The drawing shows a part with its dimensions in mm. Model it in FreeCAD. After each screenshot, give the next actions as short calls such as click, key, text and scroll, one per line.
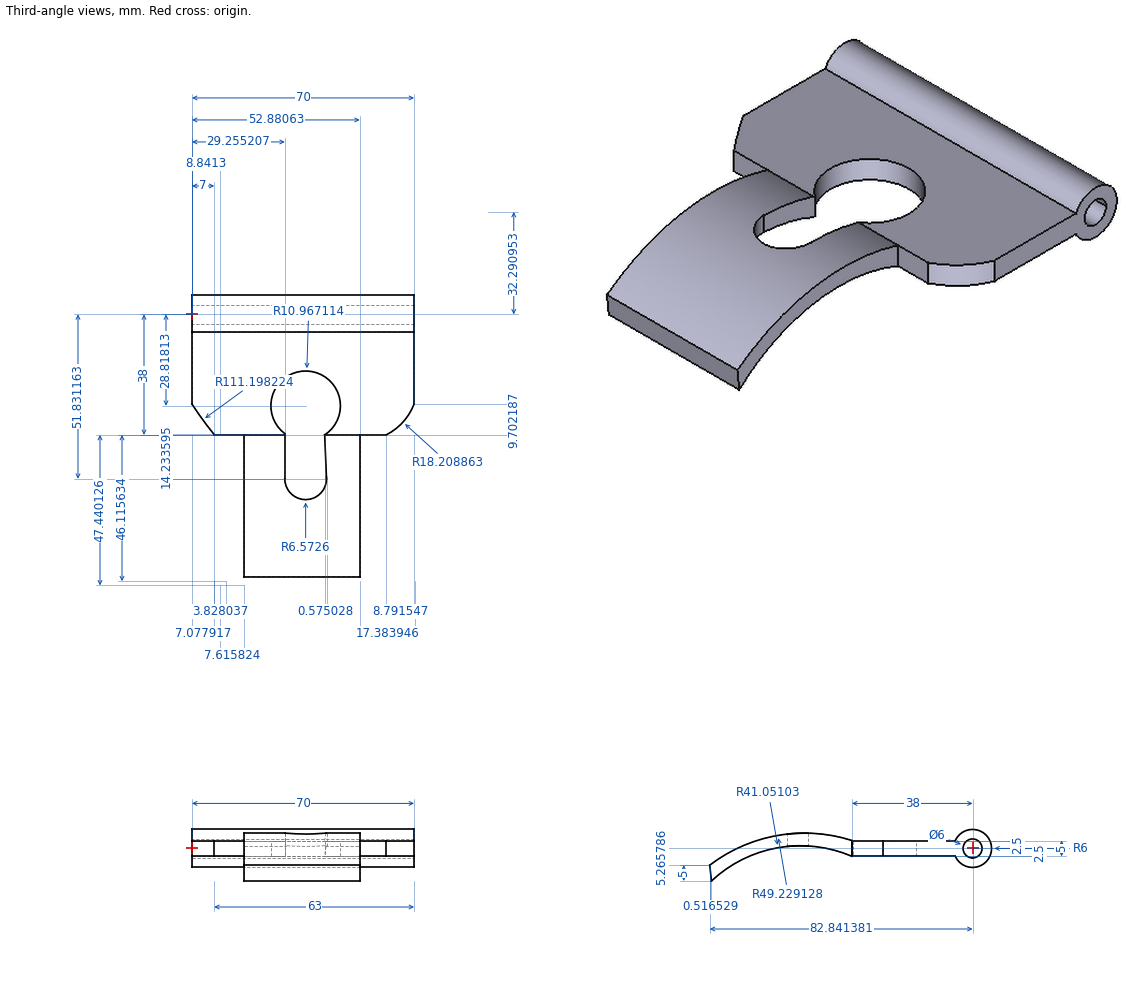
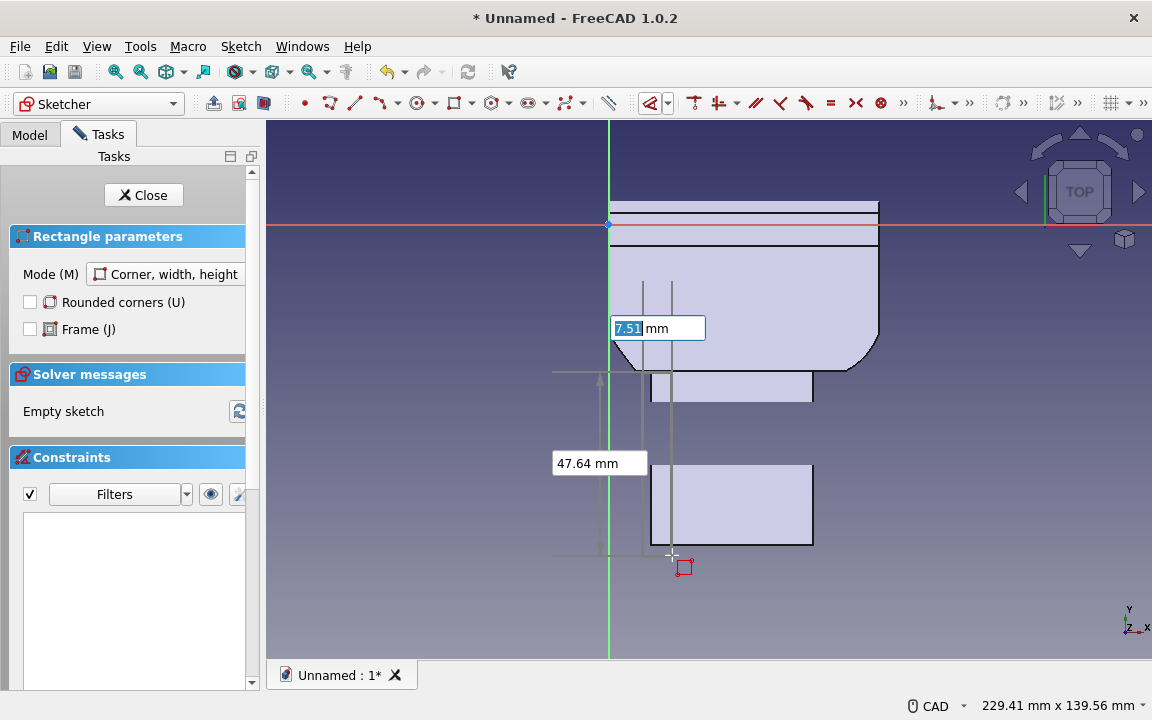
text(7.615824)
key(Tab)
text(47.440126)
key(Return)
key(Escape)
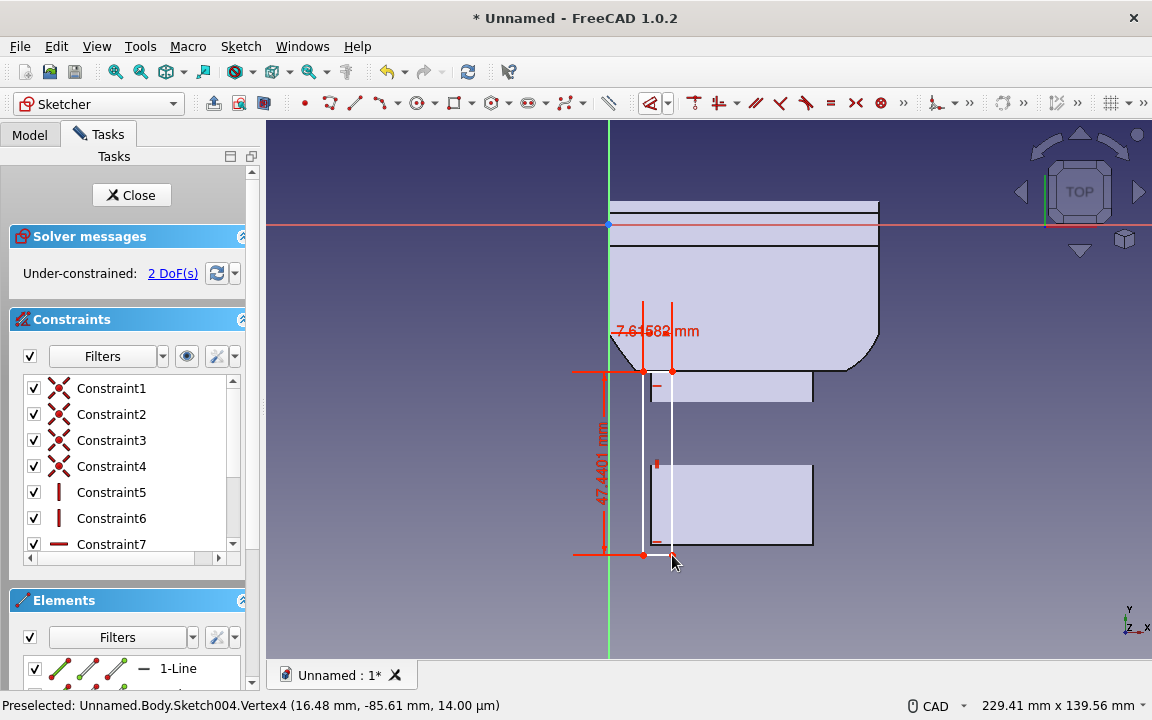
click(643, 372)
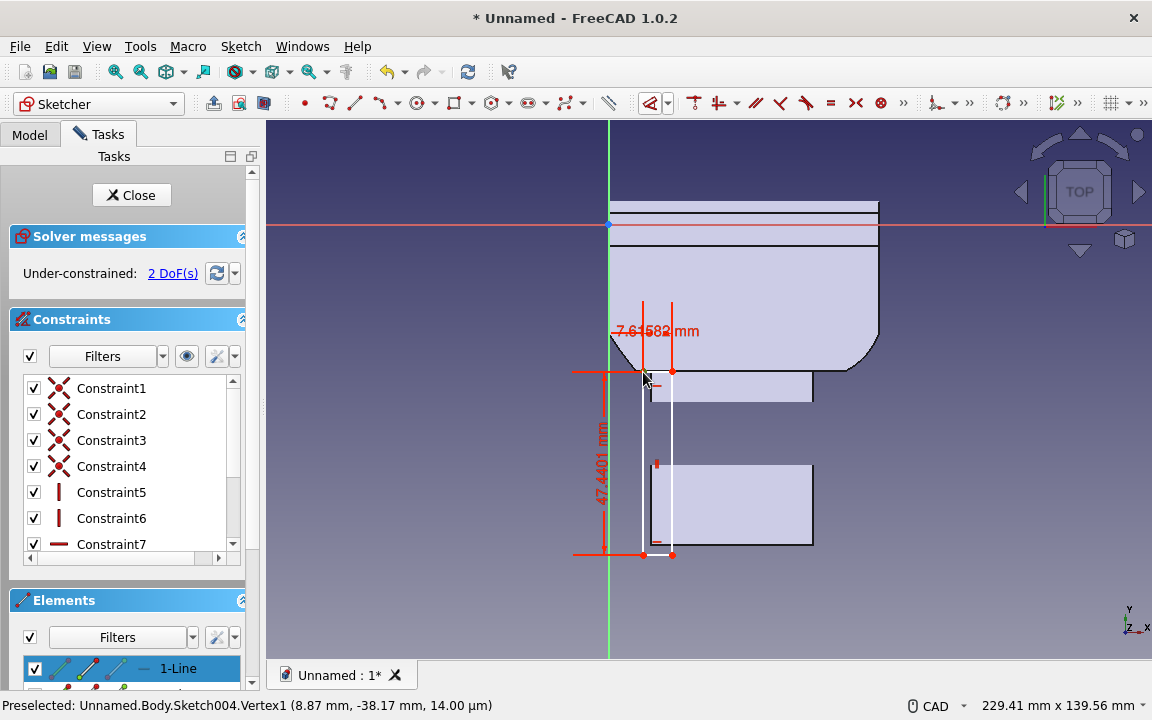
key(i)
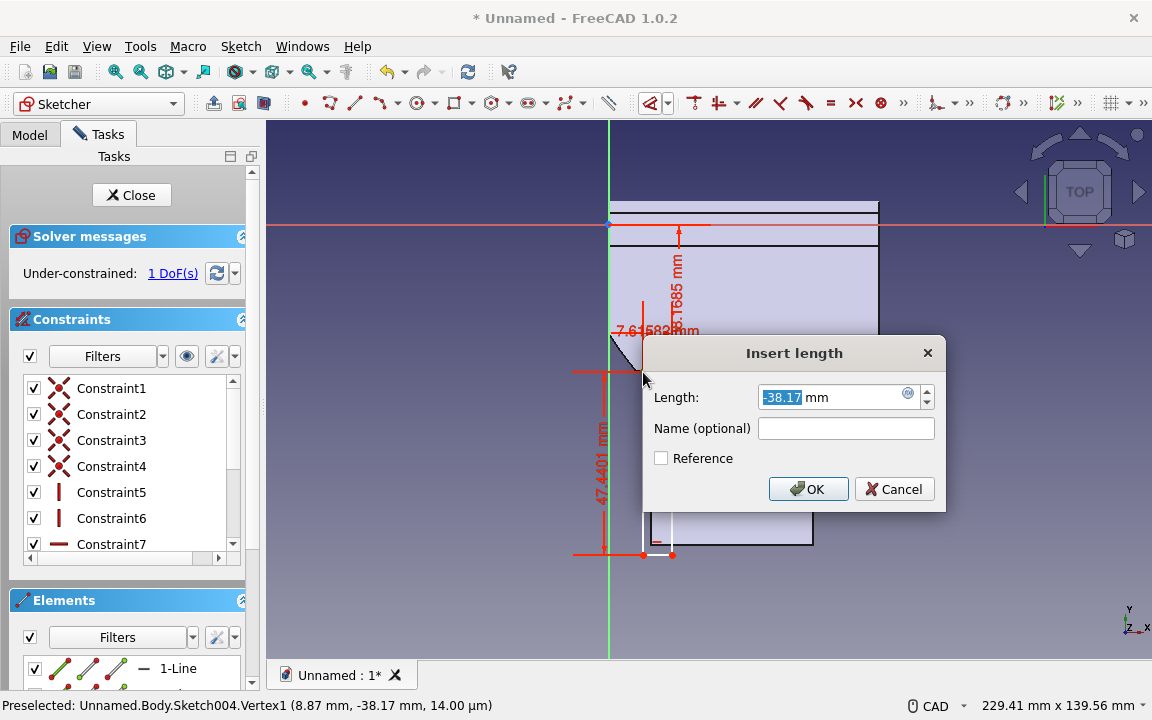
text(-38)
key(Return)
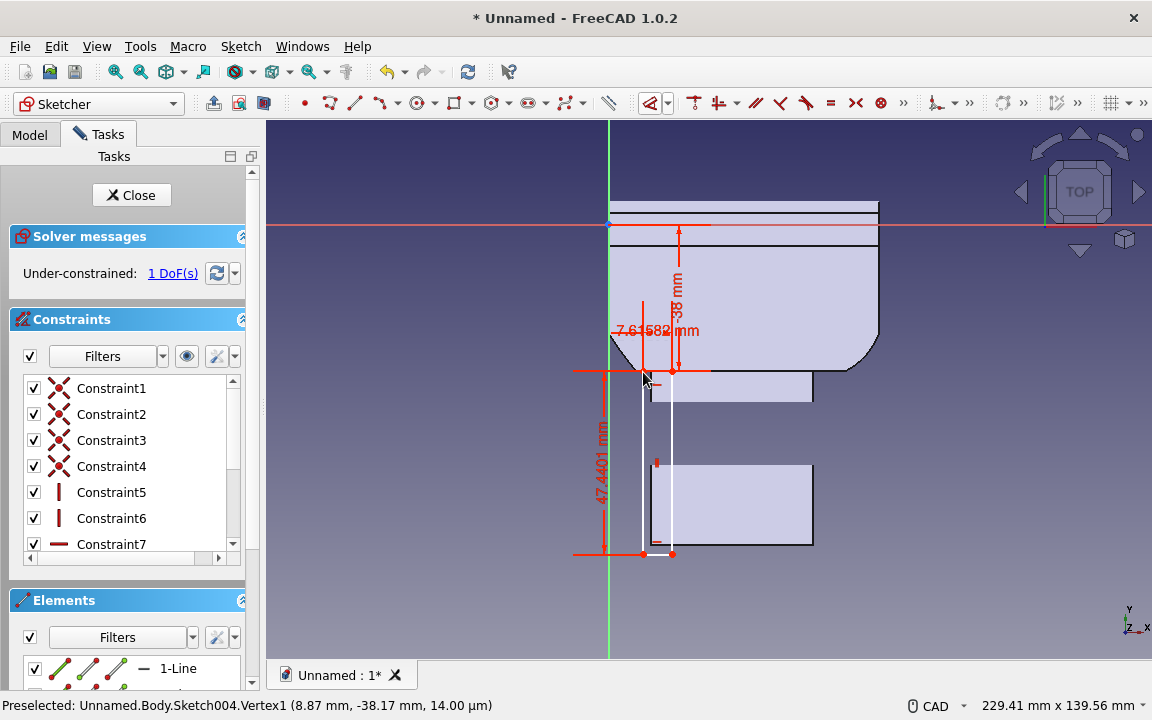
click(643, 371)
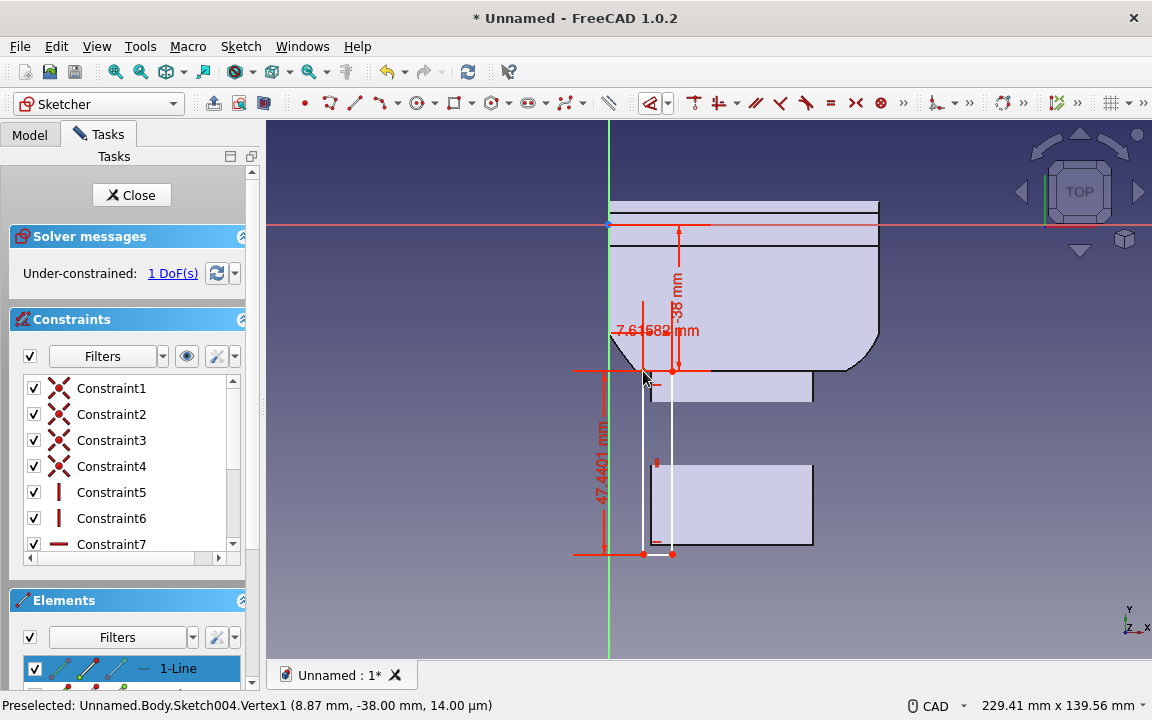
click(668, 104)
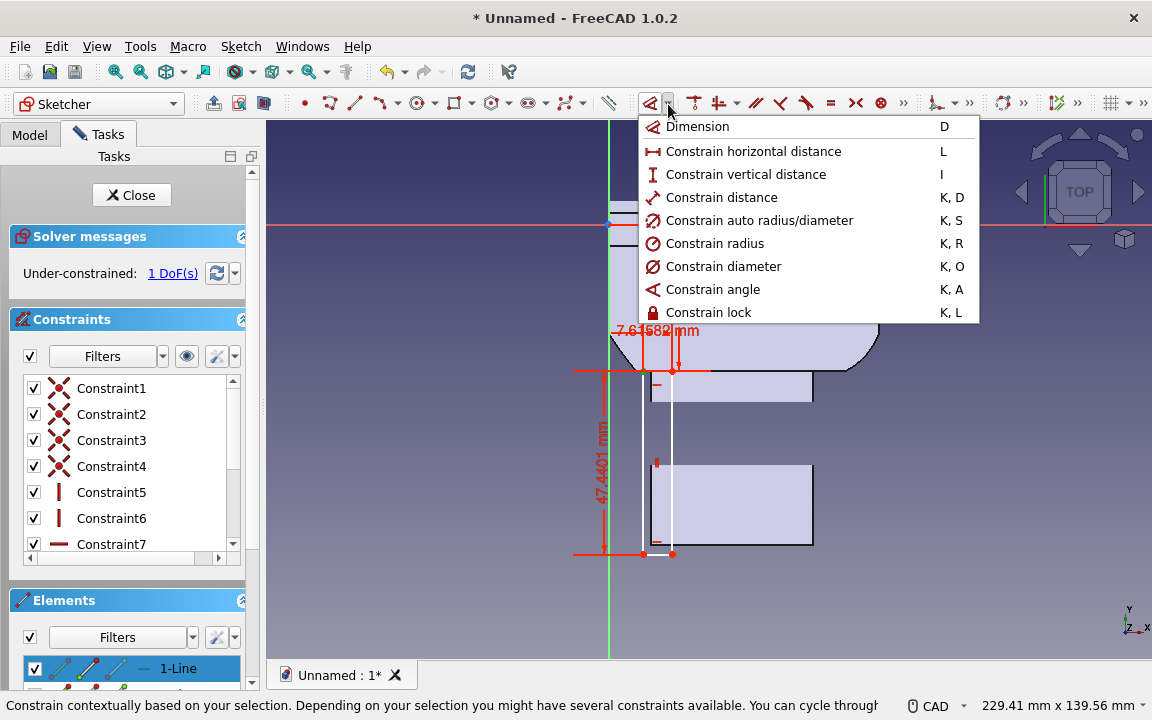
click(809, 152)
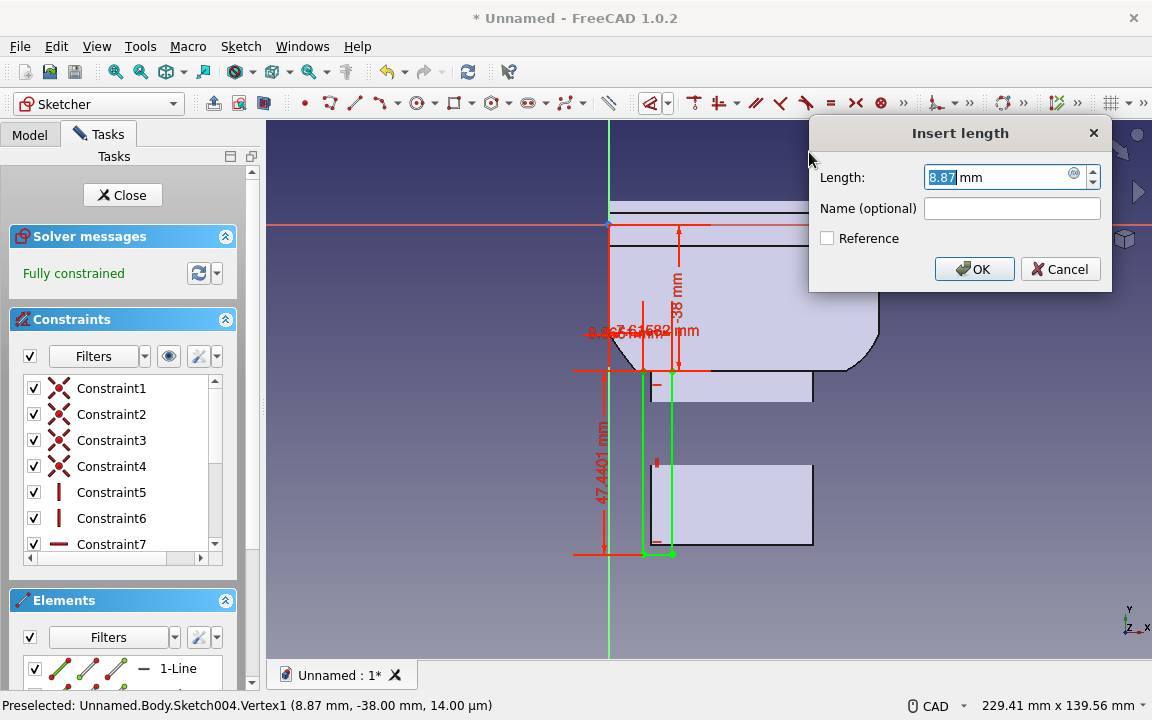
text(8.8413)
key(Return)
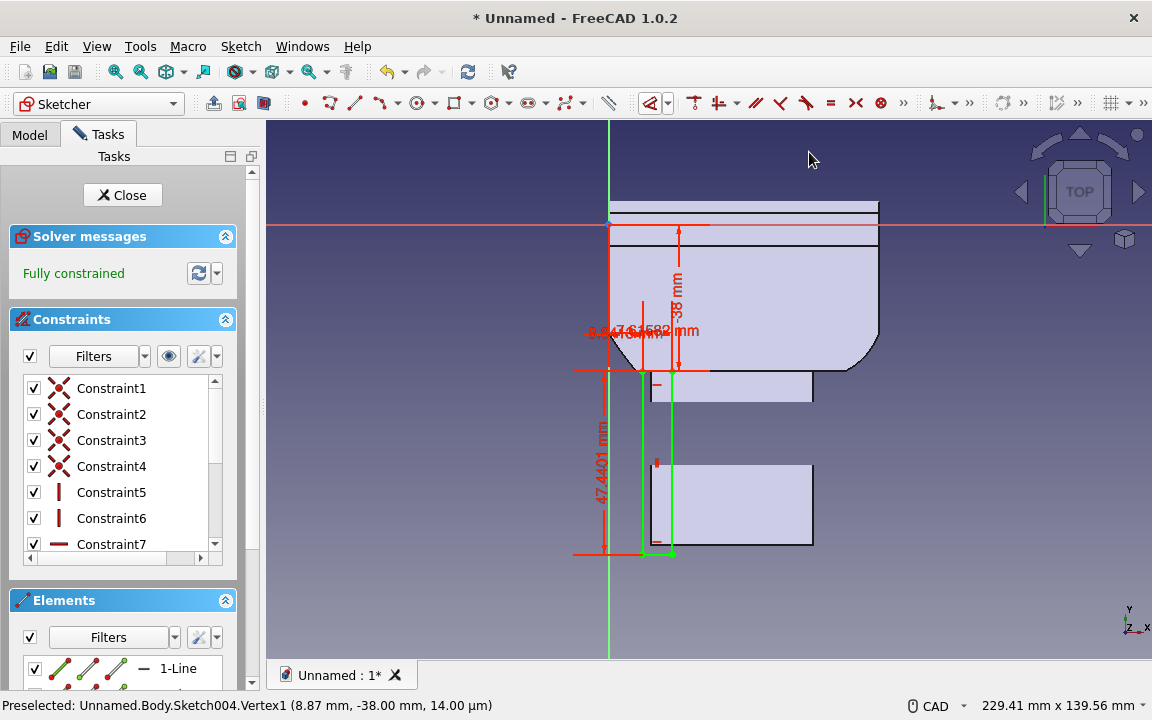
click(123, 195)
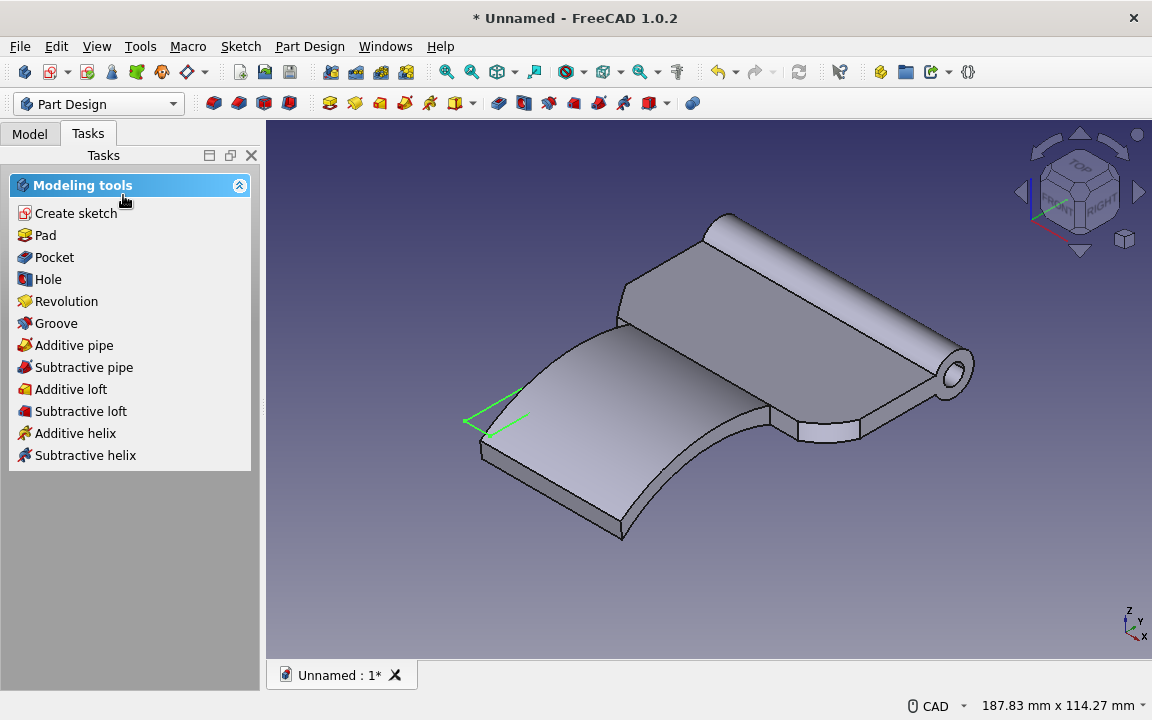
click(499, 104)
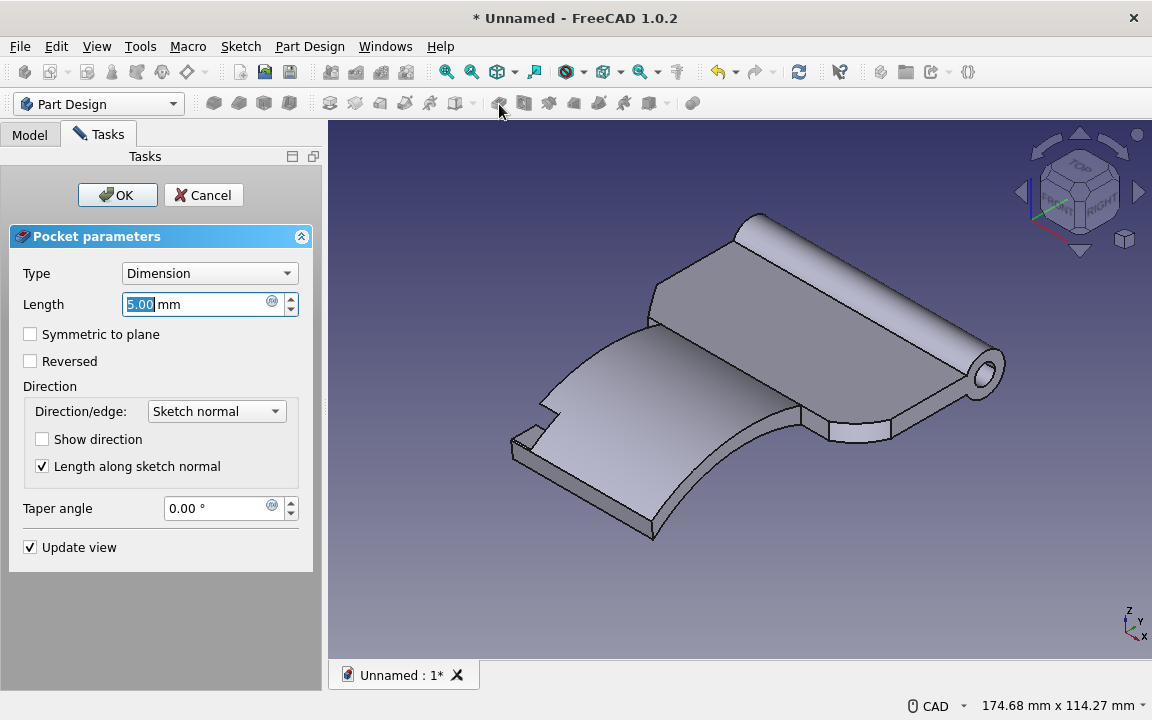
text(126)
key(Tab)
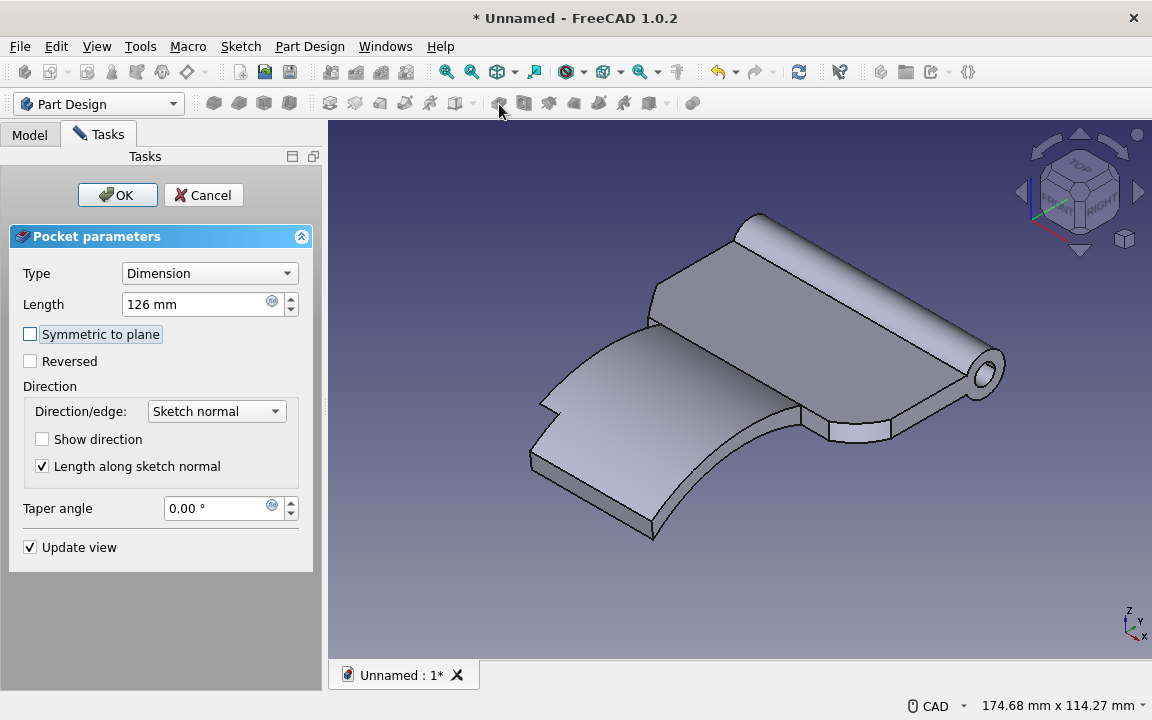
click(31, 334)